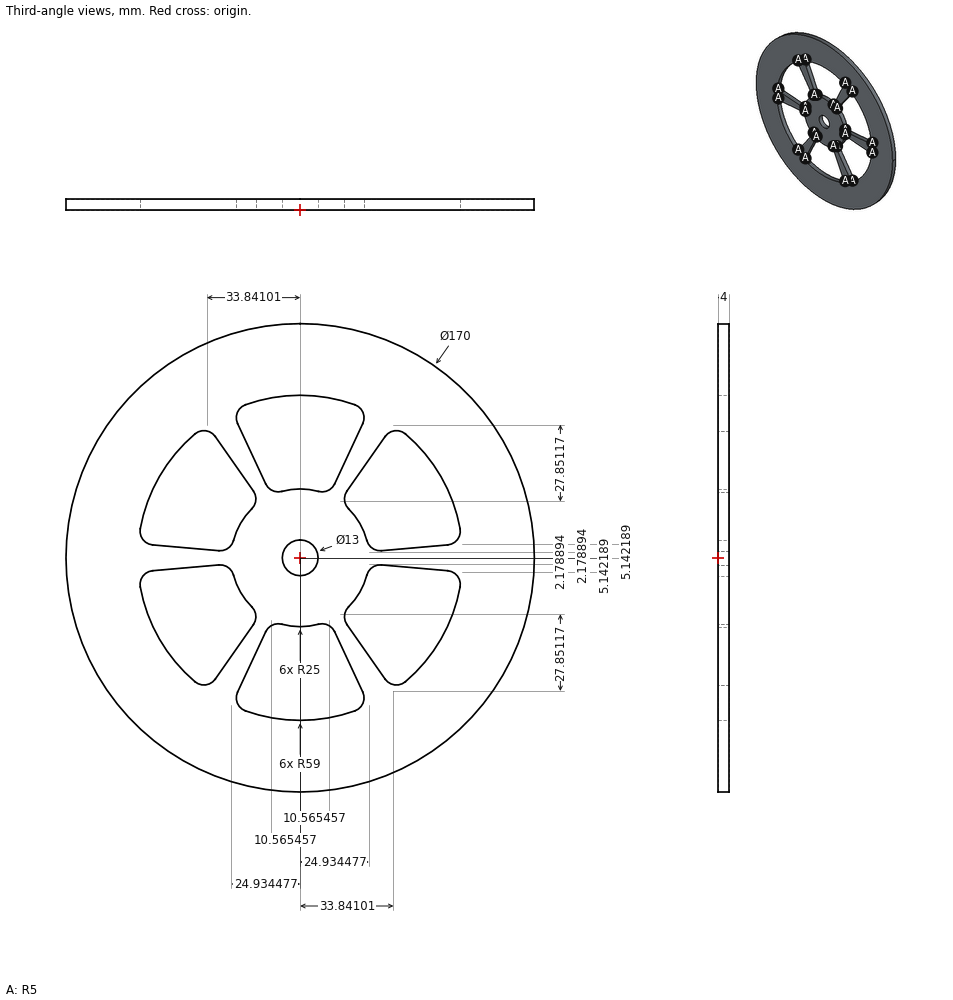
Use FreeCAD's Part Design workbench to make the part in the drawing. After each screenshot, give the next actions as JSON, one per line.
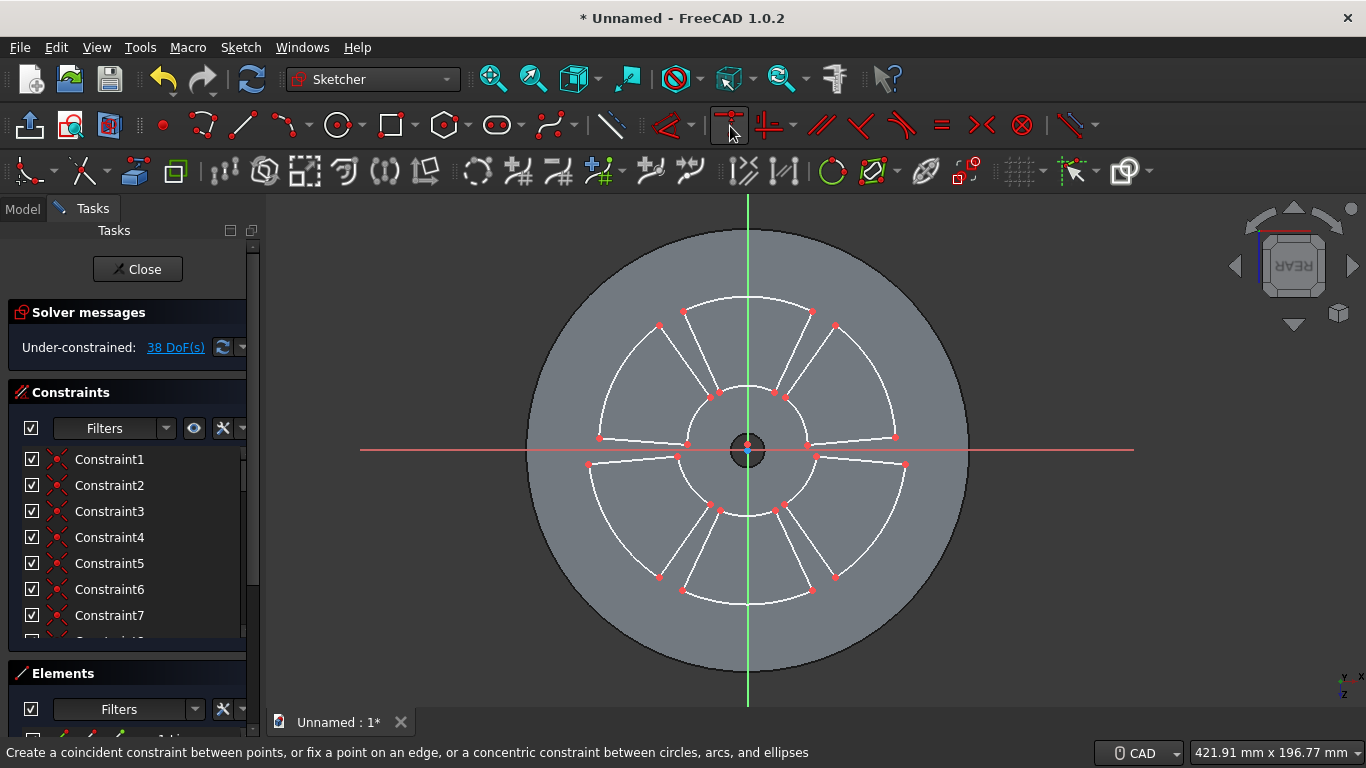
{"action": "left_click_drag", "start_coordinate": [737, 435], "coordinate": [758, 460]}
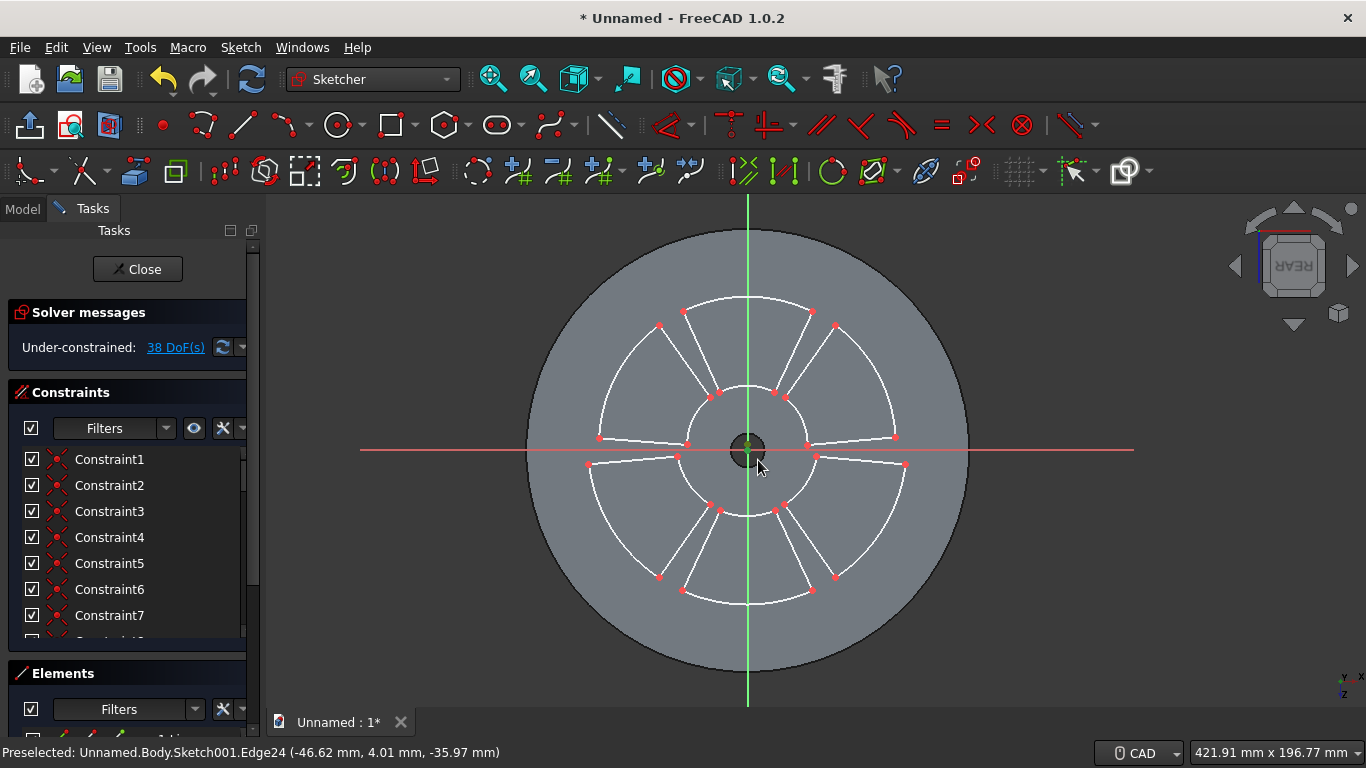
{"action": "left_click", "coordinate": [730, 126]}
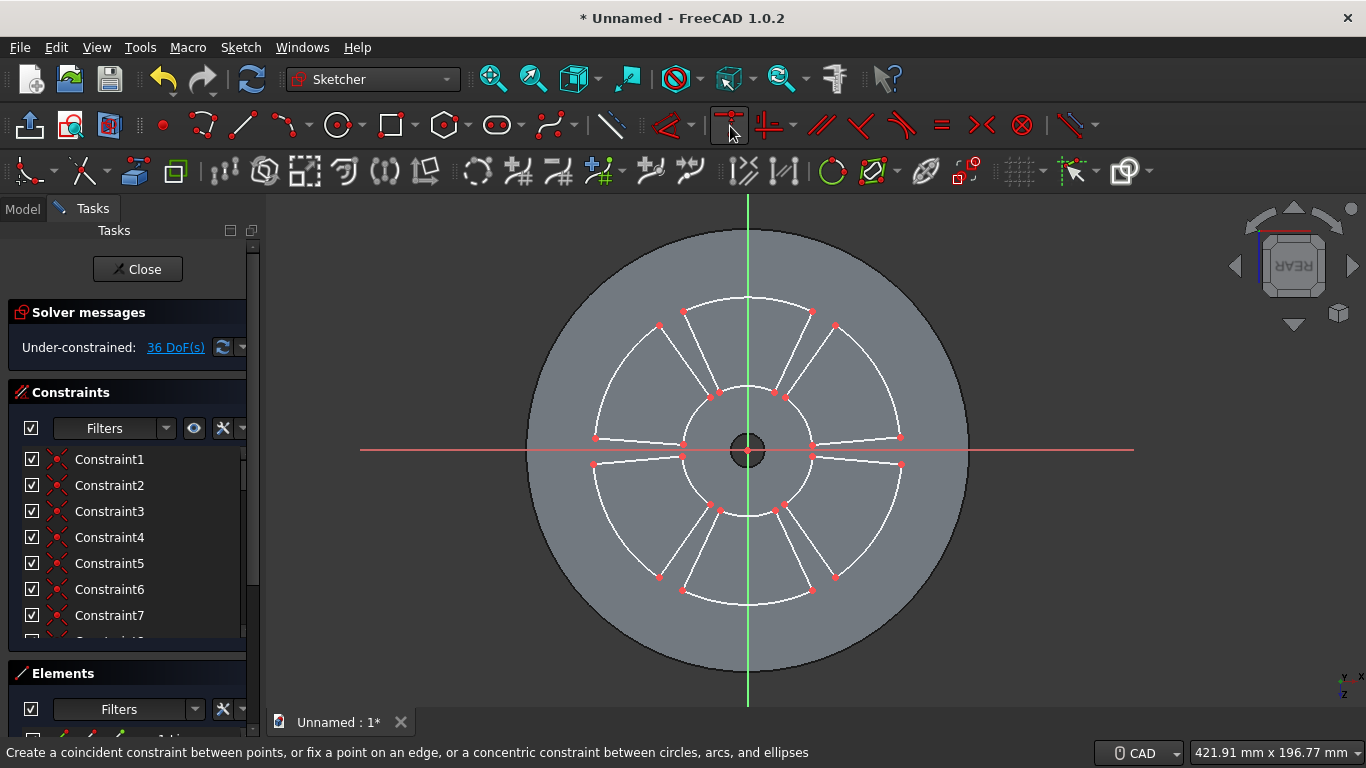
{"action": "scroll", "coordinate": [759, 387], "scroll_direction": "up", "scroll_amount": 2}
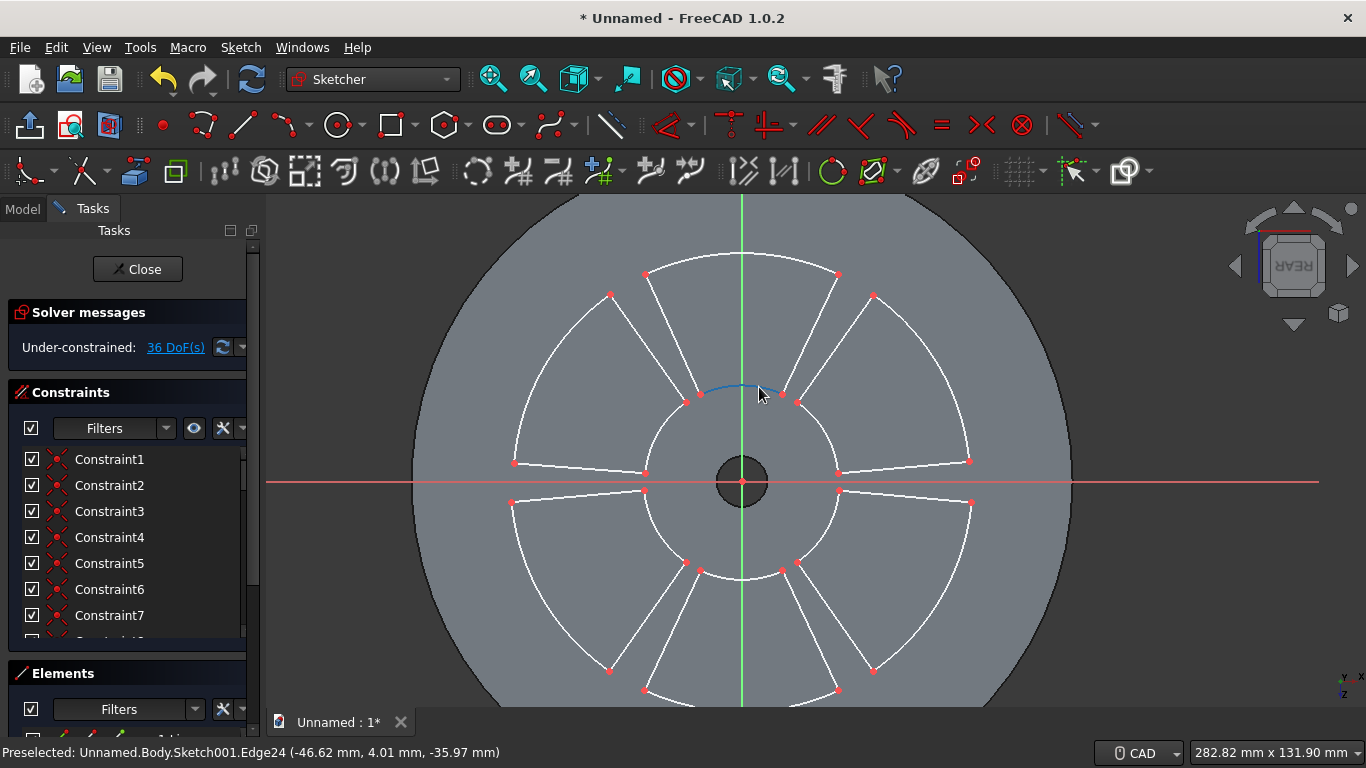
{"action": "left_click", "coordinate": [758, 387]}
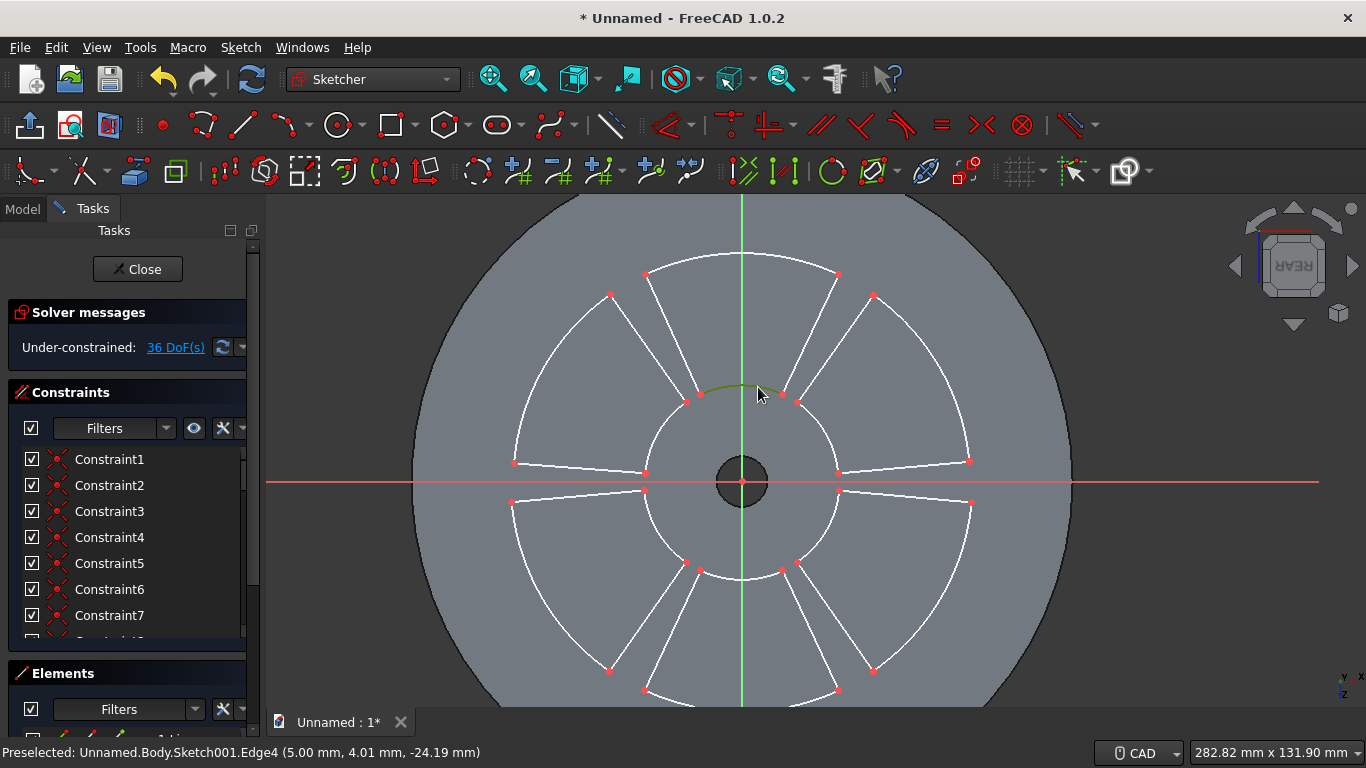
{"action": "left_click", "coordinate": [833, 449]}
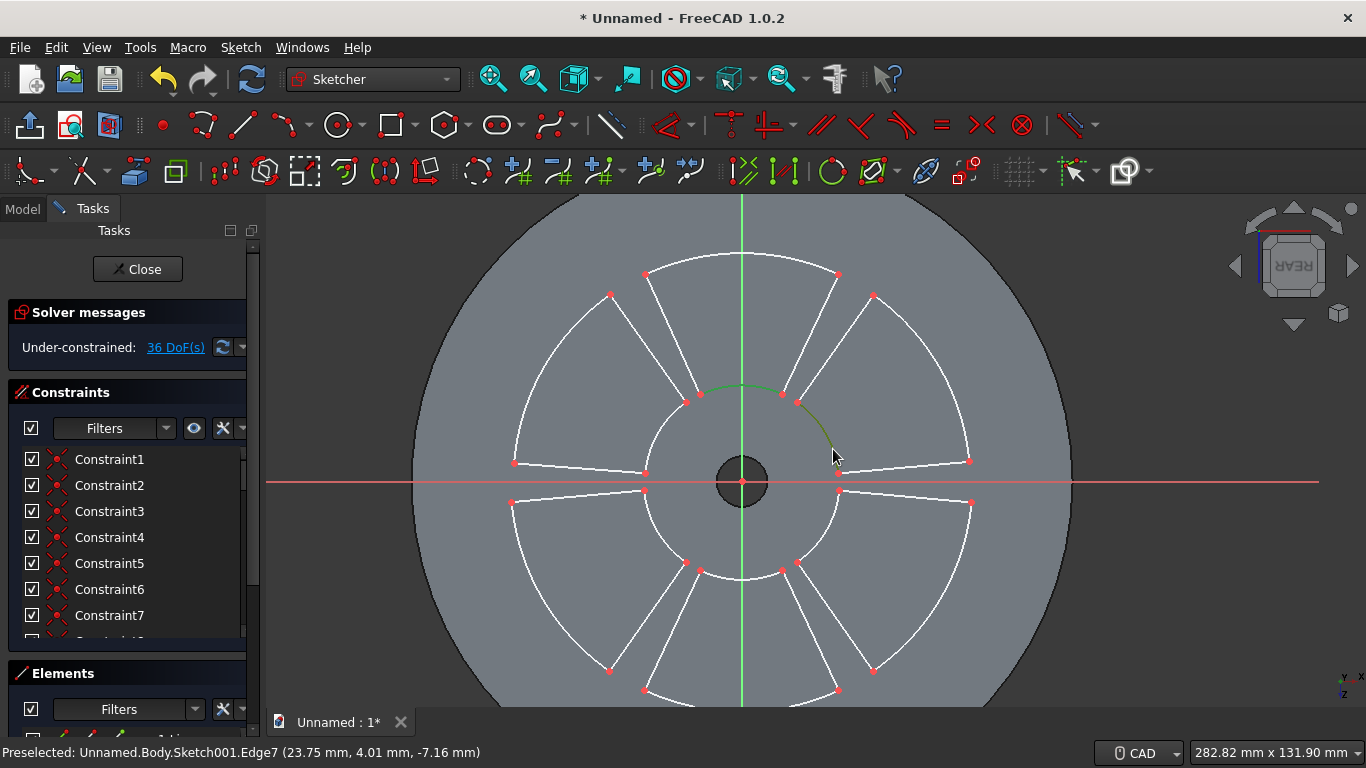
{"action": "left_click", "coordinate": [816, 545]}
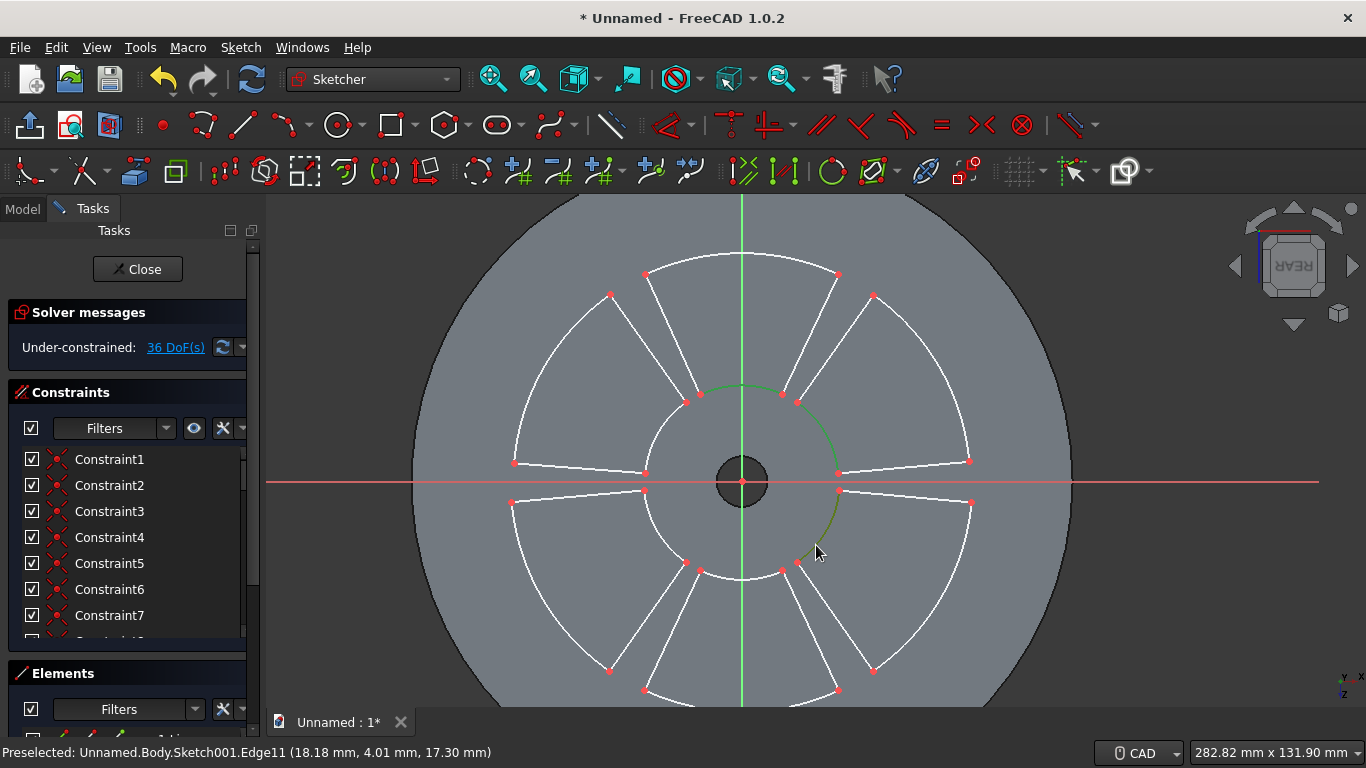
{"action": "left_click", "coordinate": [725, 578]}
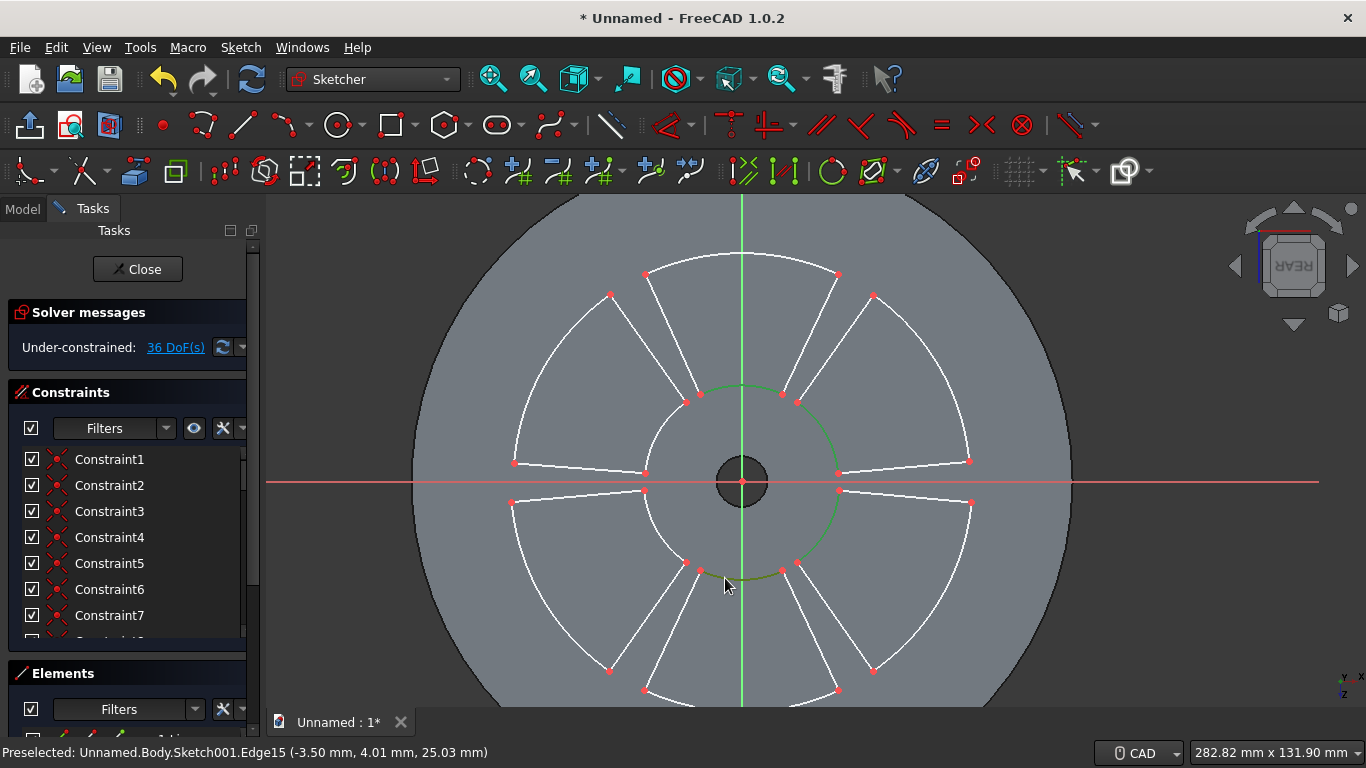
{"action": "left_click", "coordinate": [650, 515]}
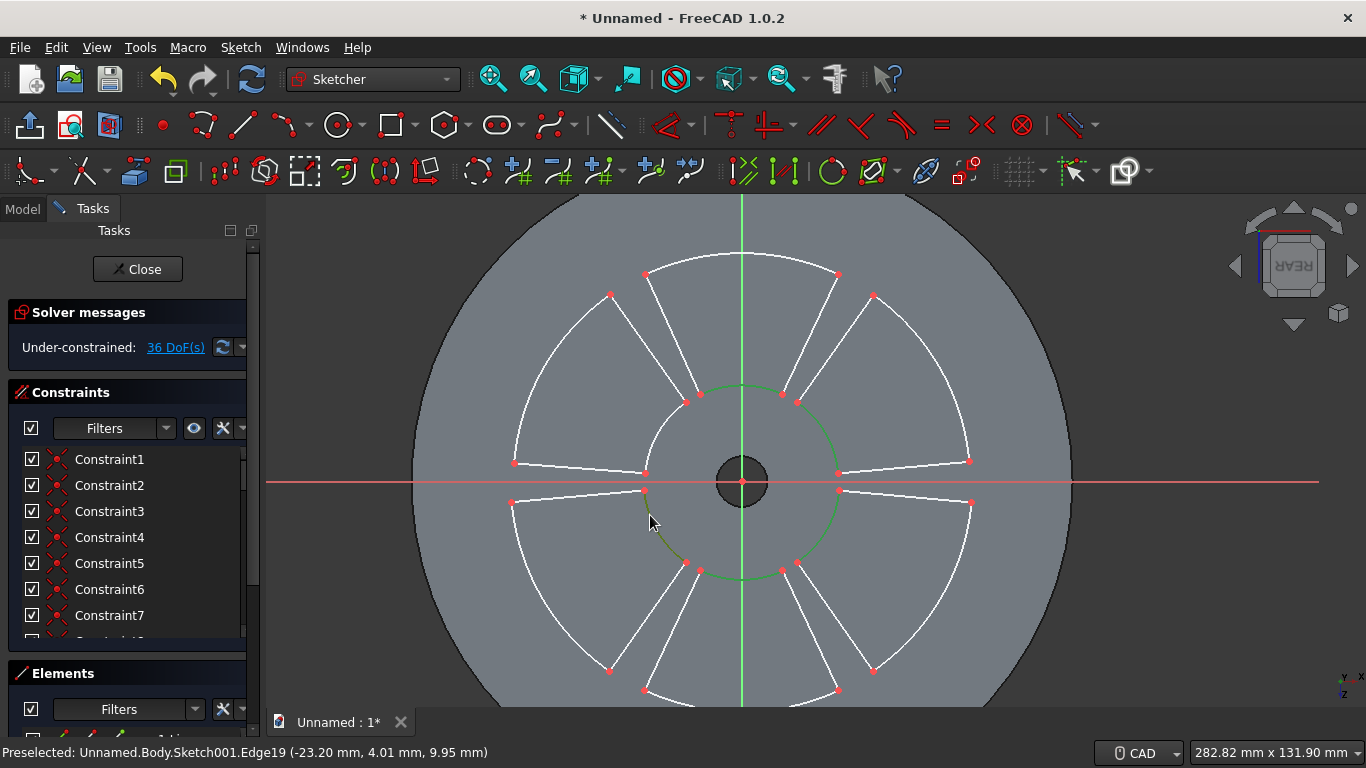
{"action": "left_click", "coordinate": [668, 419]}